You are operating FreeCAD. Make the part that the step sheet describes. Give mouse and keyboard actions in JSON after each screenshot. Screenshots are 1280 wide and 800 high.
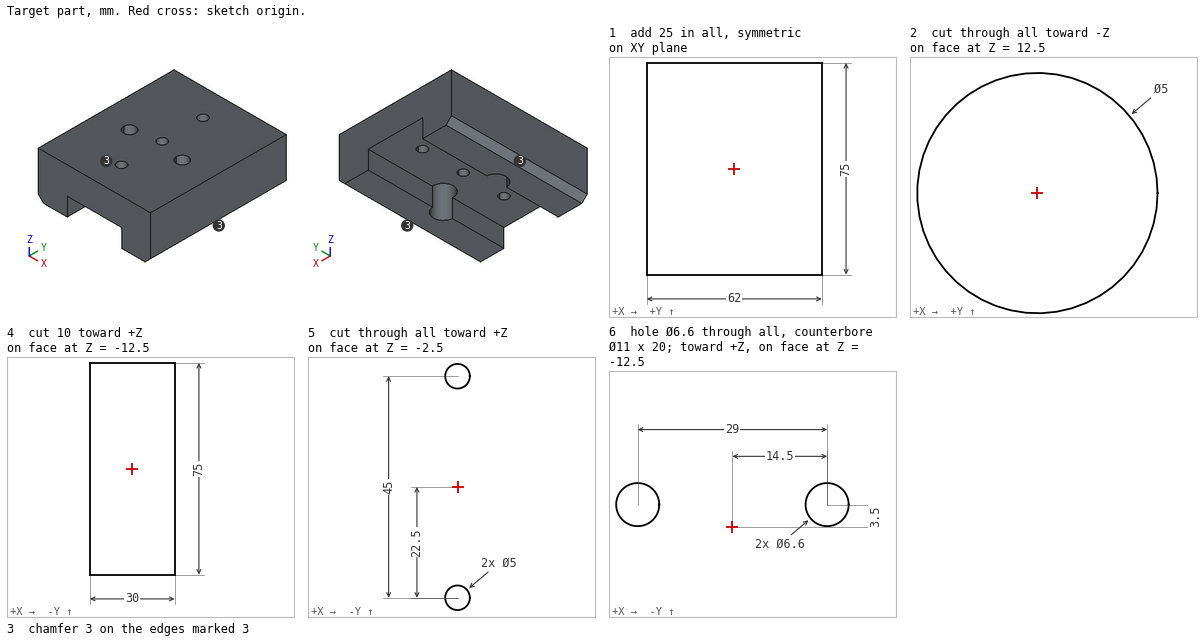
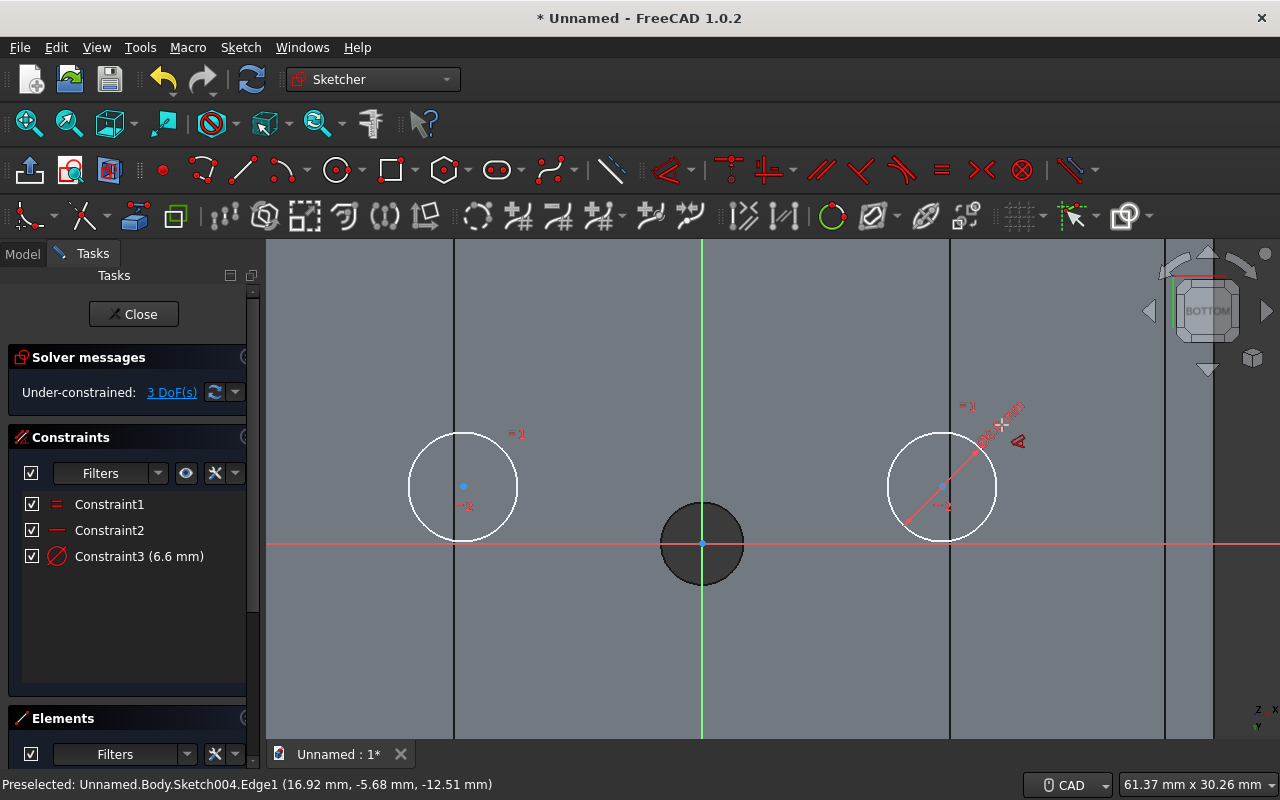
{"action": "left_click", "coordinate": [942, 487]}
{"action": "left_click", "coordinate": [976, 502]}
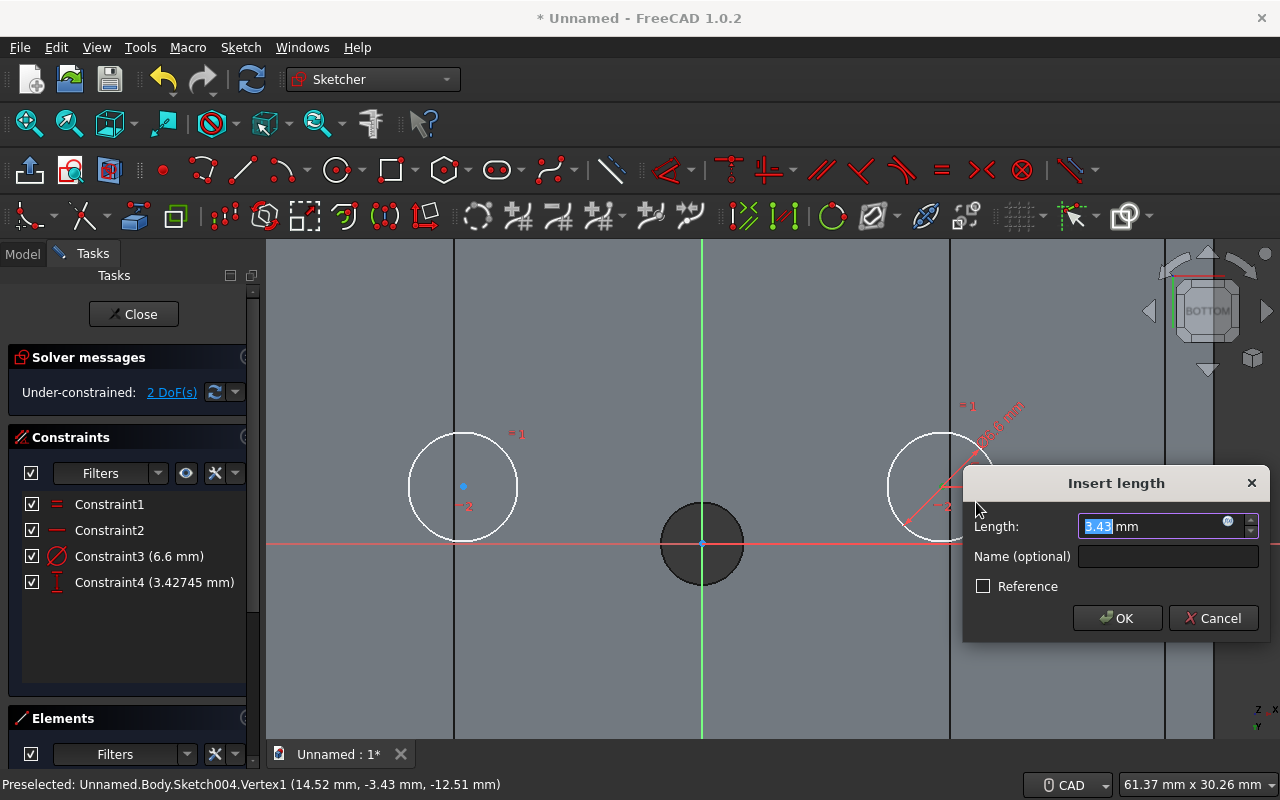
{"action": "type", "text": "3.5"}
{"action": "key", "text": "Return"}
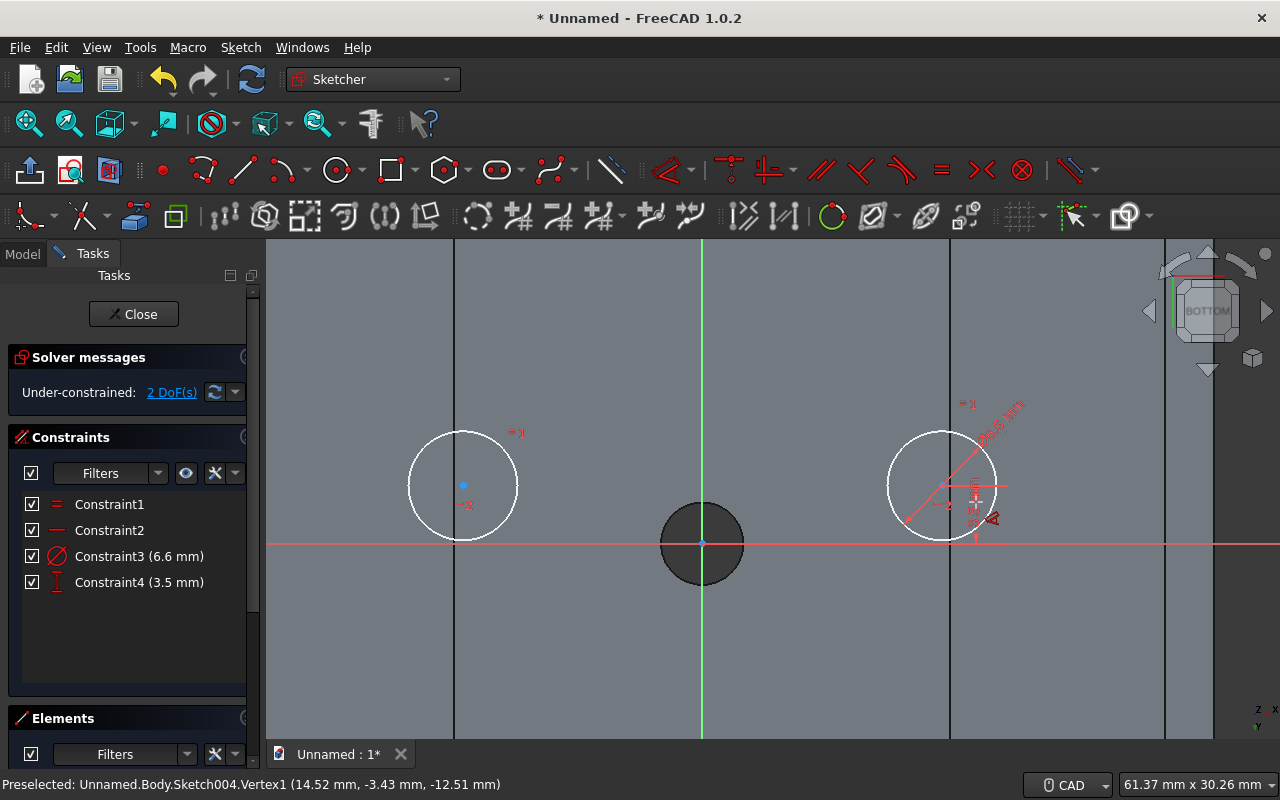
{"action": "left_click", "coordinate": [942, 486]}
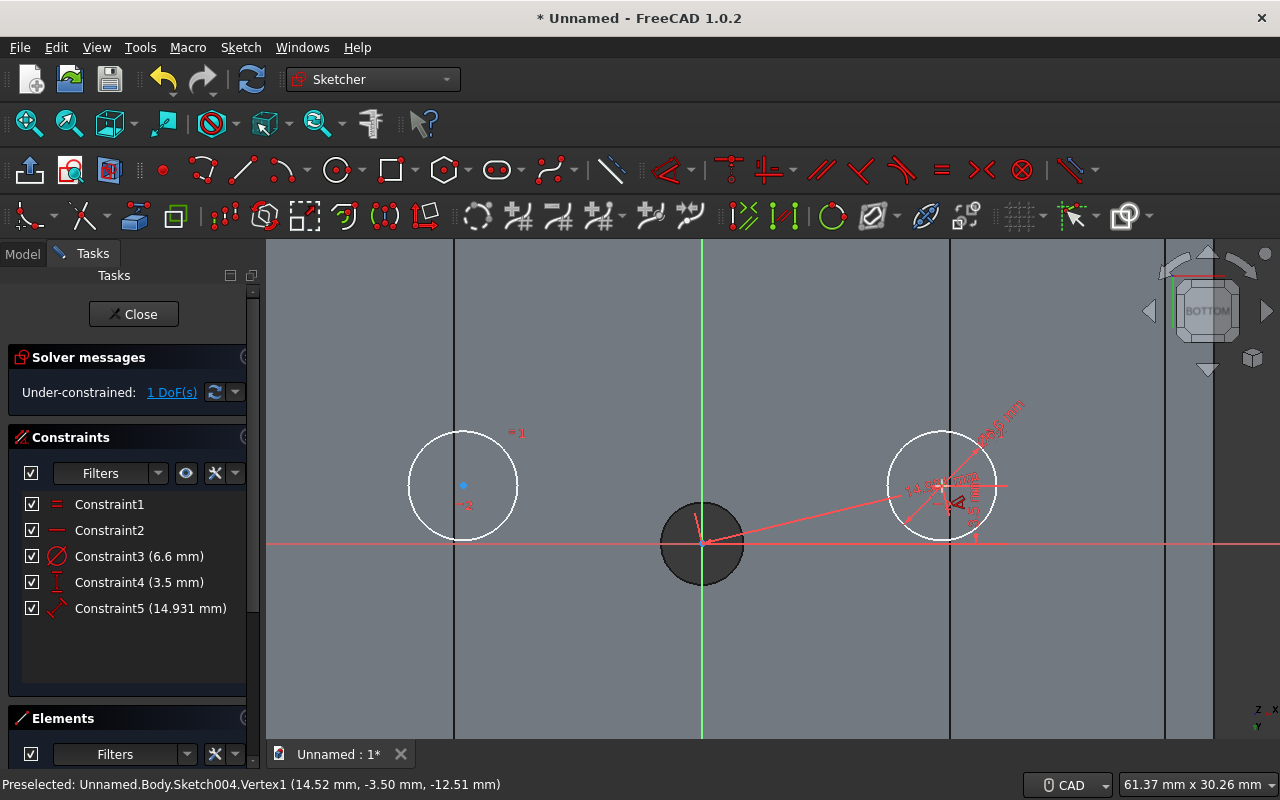
{"action": "left_click", "coordinate": [463, 486]}
{"action": "left_click", "coordinate": [592, 452]}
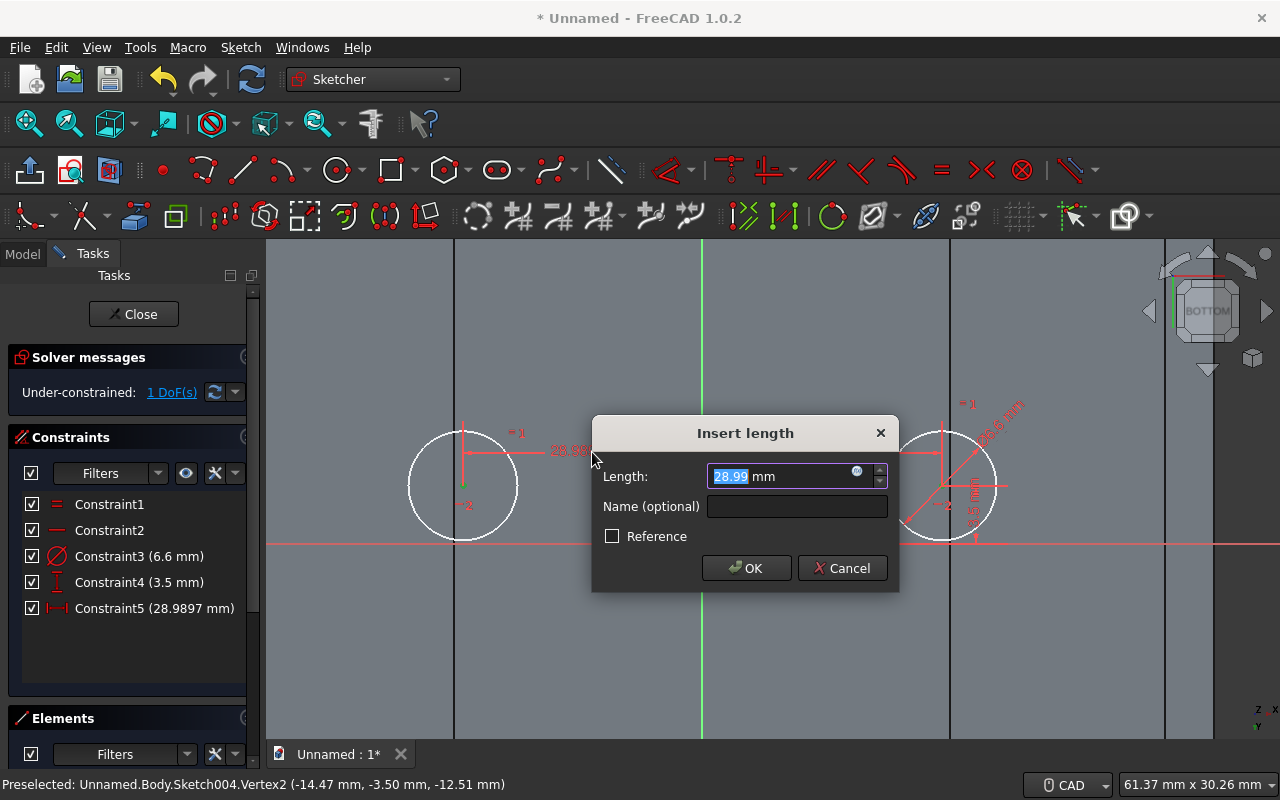
{"action": "type", "text": "29"}
{"action": "key", "text": "Return"}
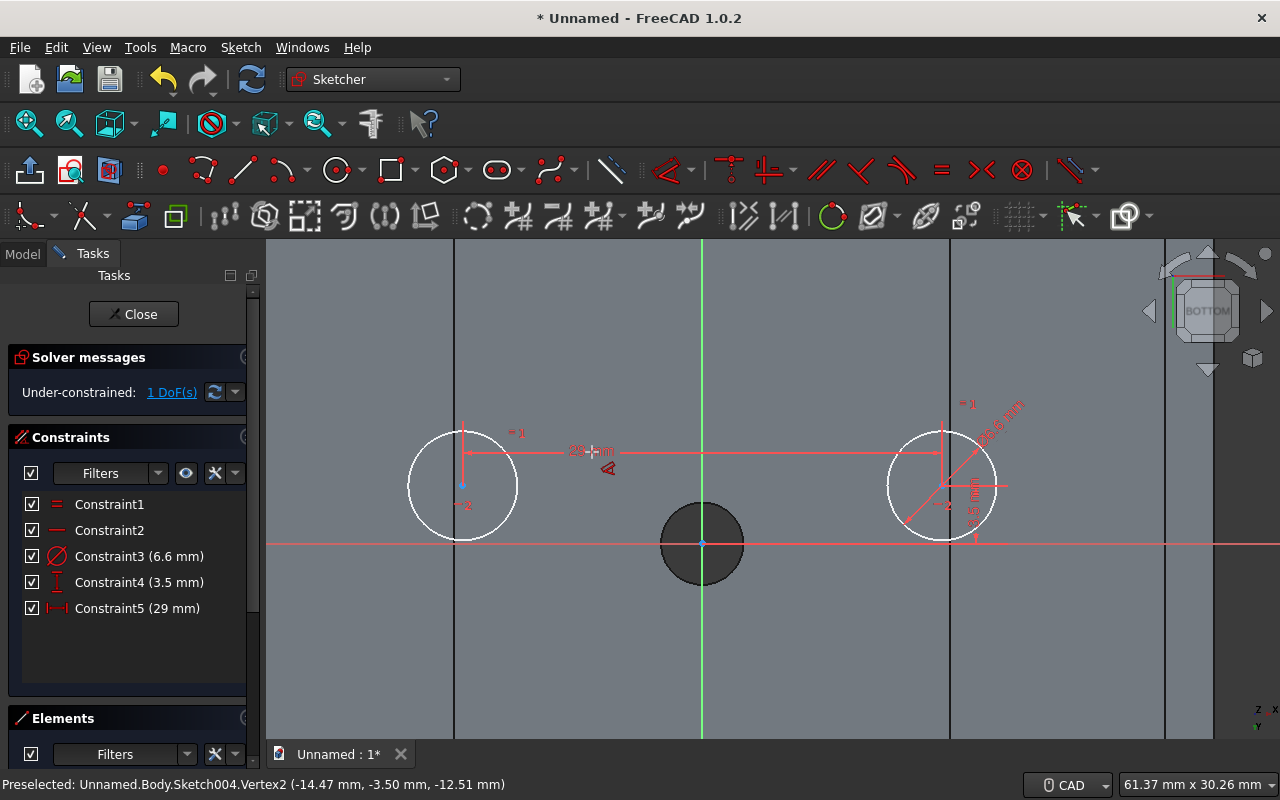
{"action": "left_click", "coordinate": [942, 486]}
{"action": "left_click", "coordinate": [822, 578]}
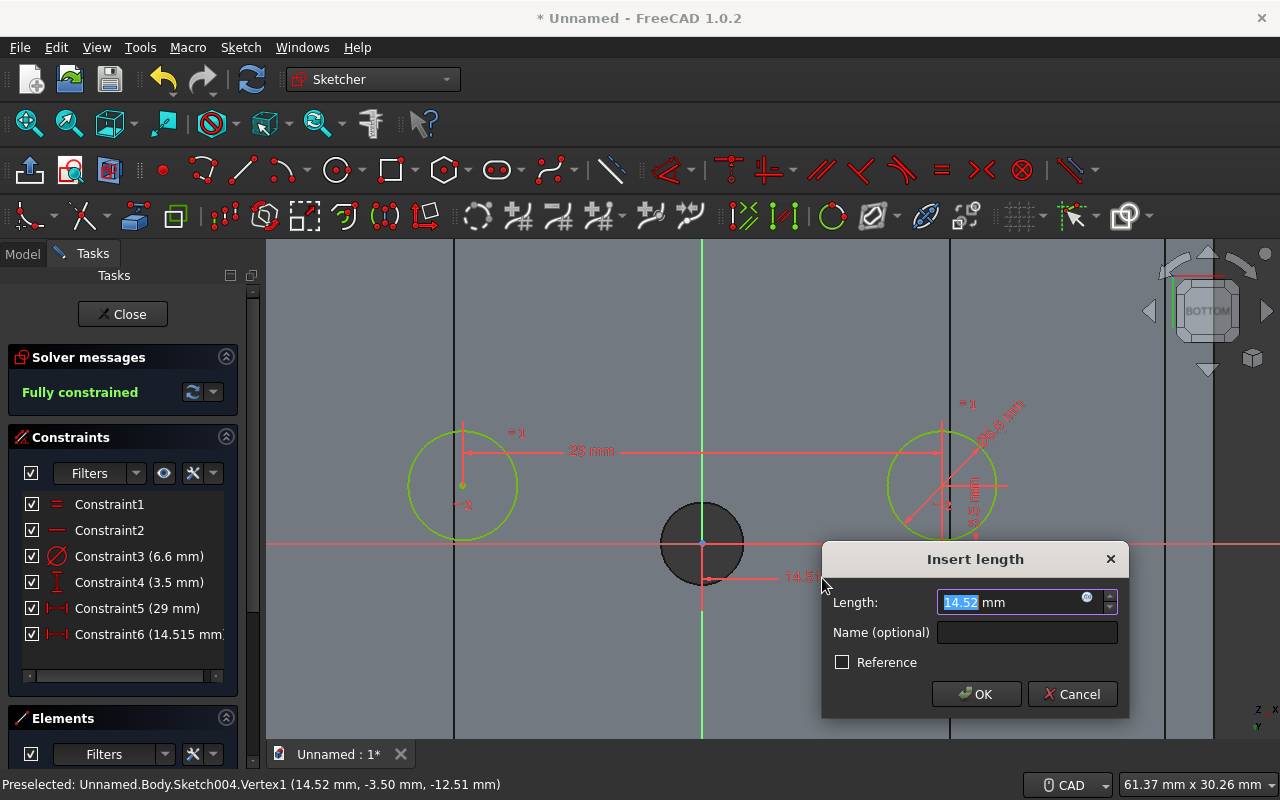
{"action": "type", "text": "14.5"}
{"action": "key", "text": "Return"}
{"action": "key", "text": "Escape"}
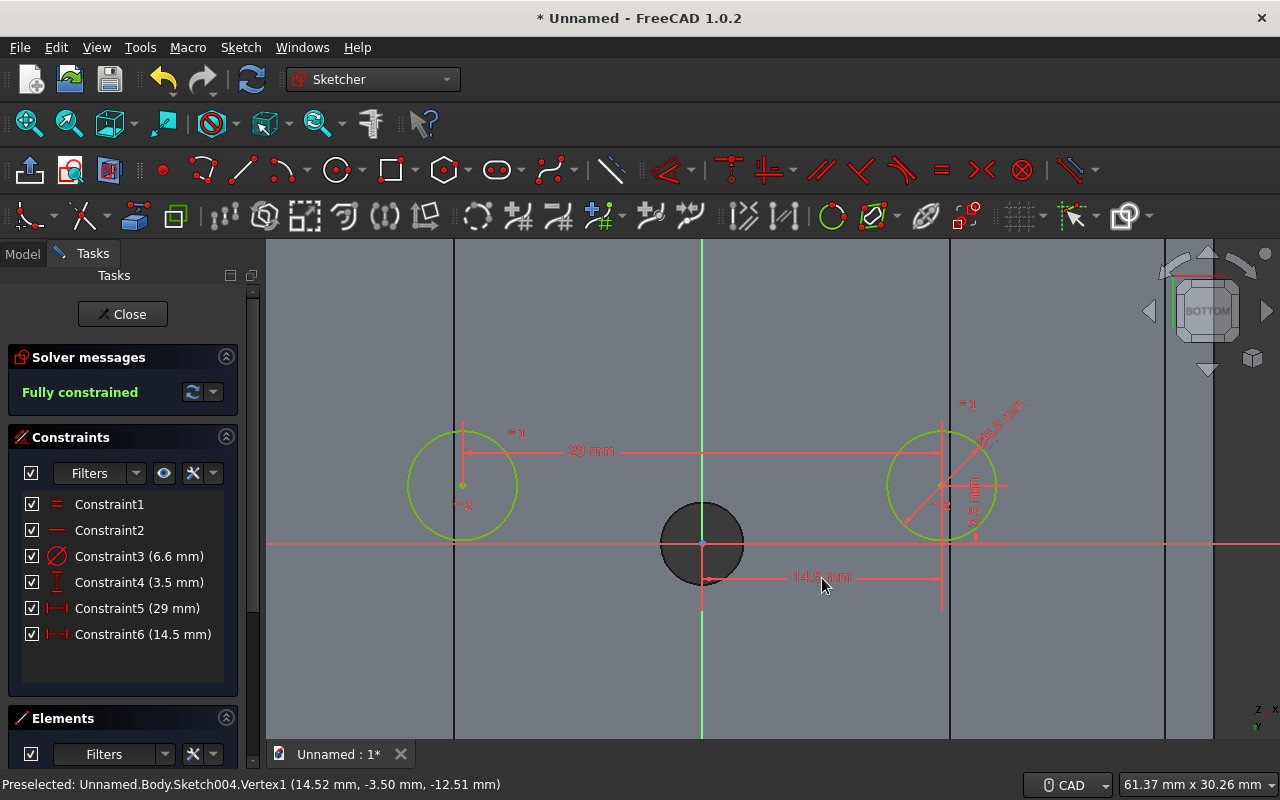
{"action": "left_click", "coordinate": [123, 314]}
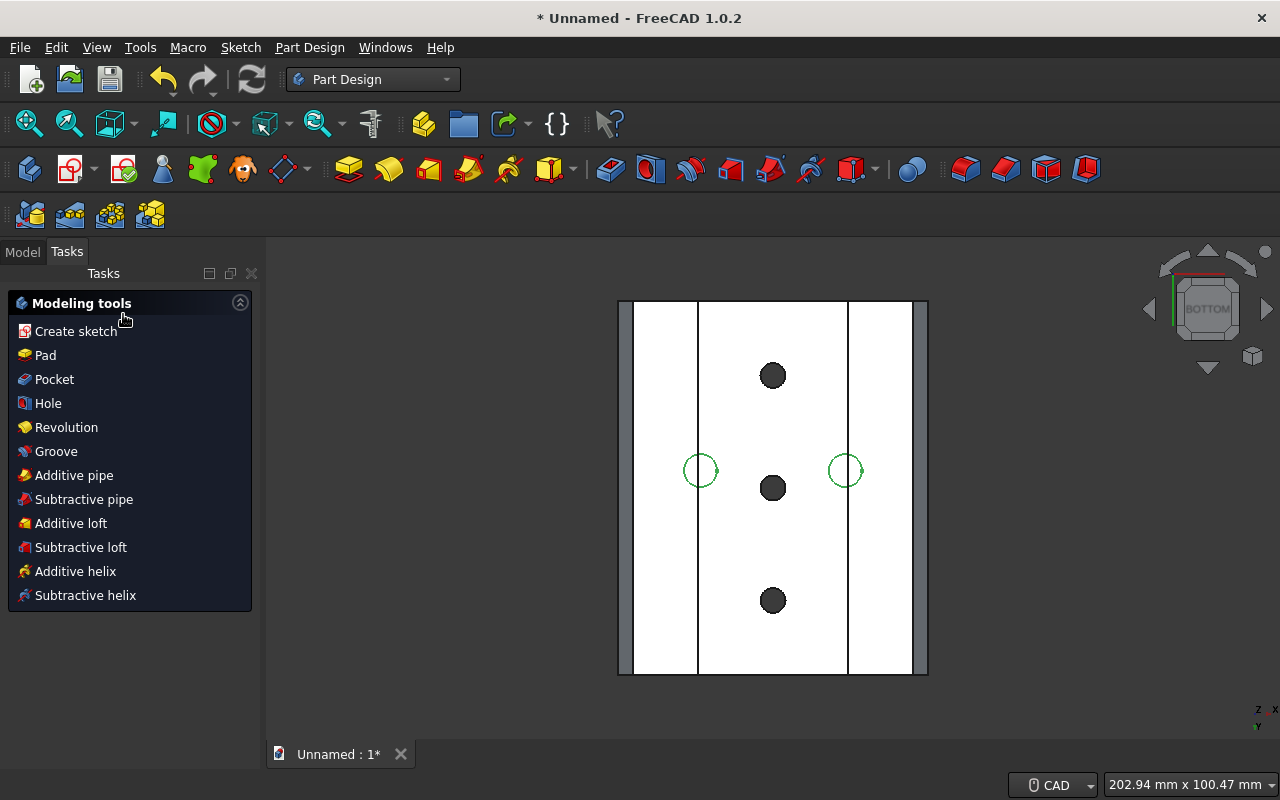
{"action": "left_click", "coordinate": [652, 170]}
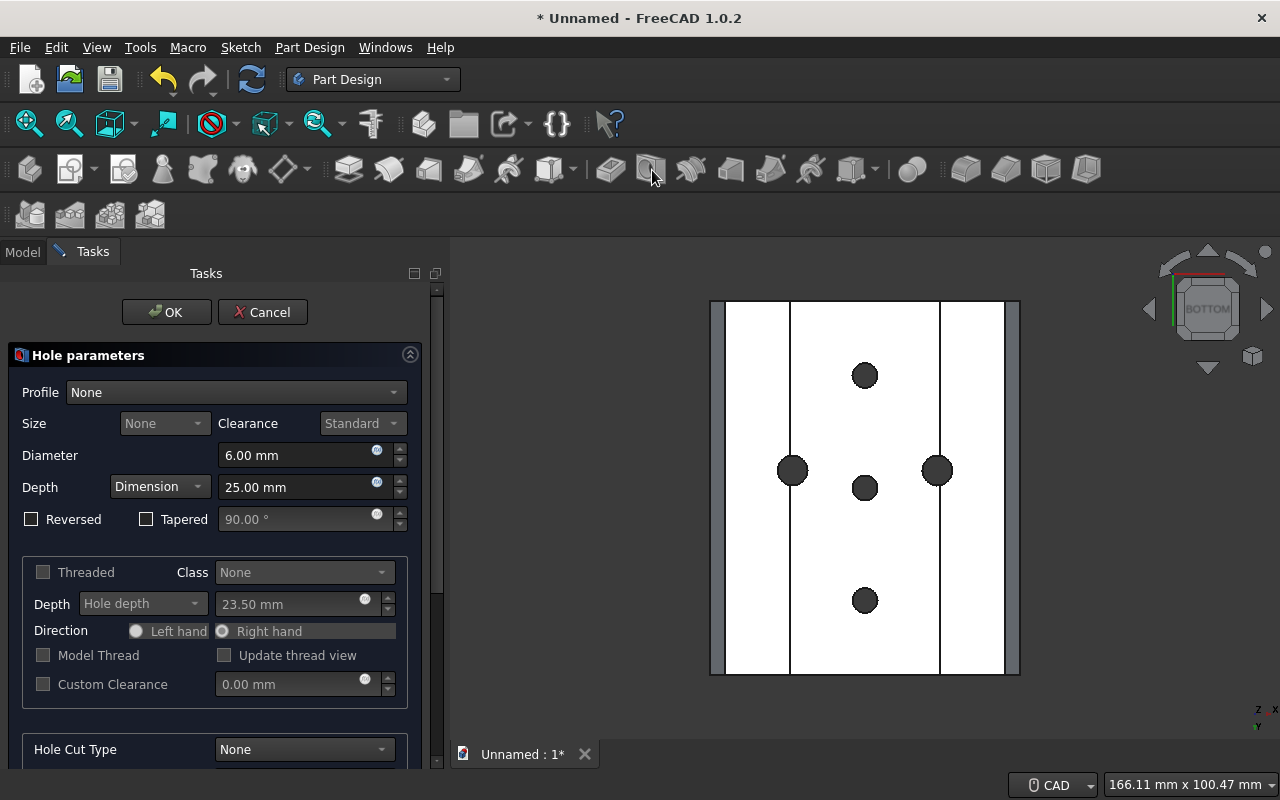
{"action": "triple_click", "coordinate": [305, 455]}